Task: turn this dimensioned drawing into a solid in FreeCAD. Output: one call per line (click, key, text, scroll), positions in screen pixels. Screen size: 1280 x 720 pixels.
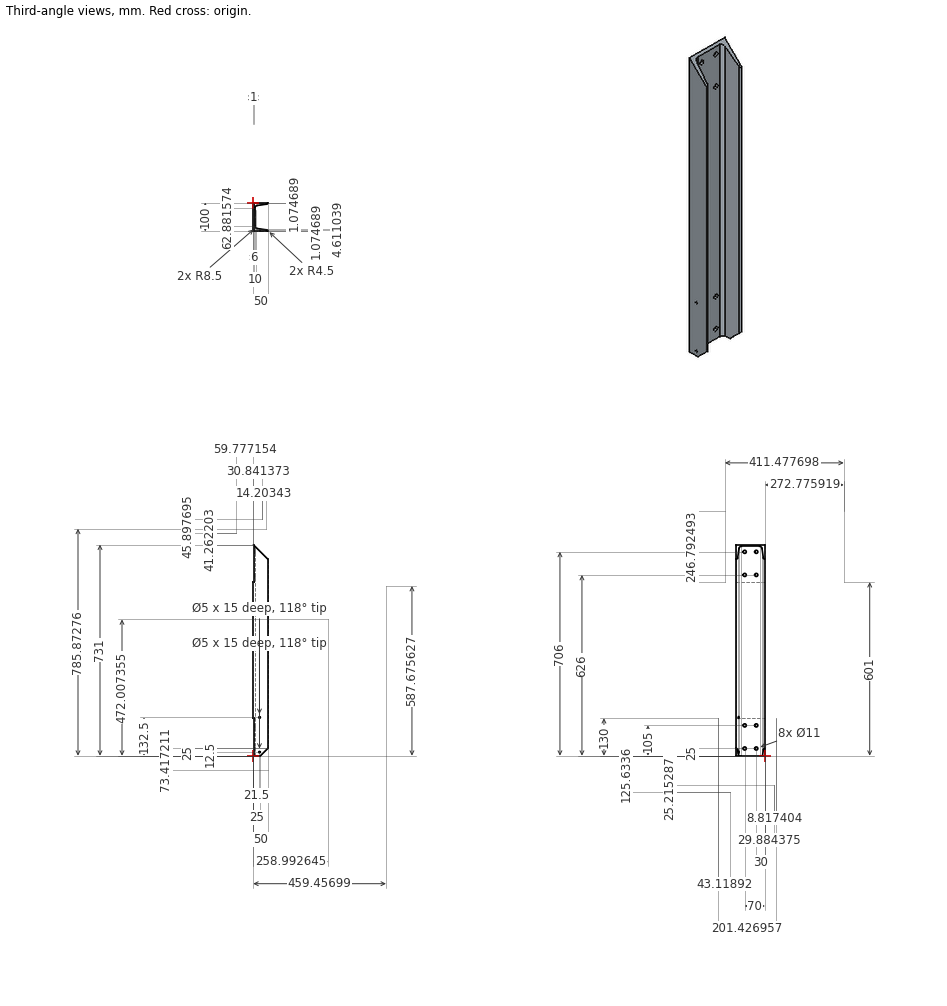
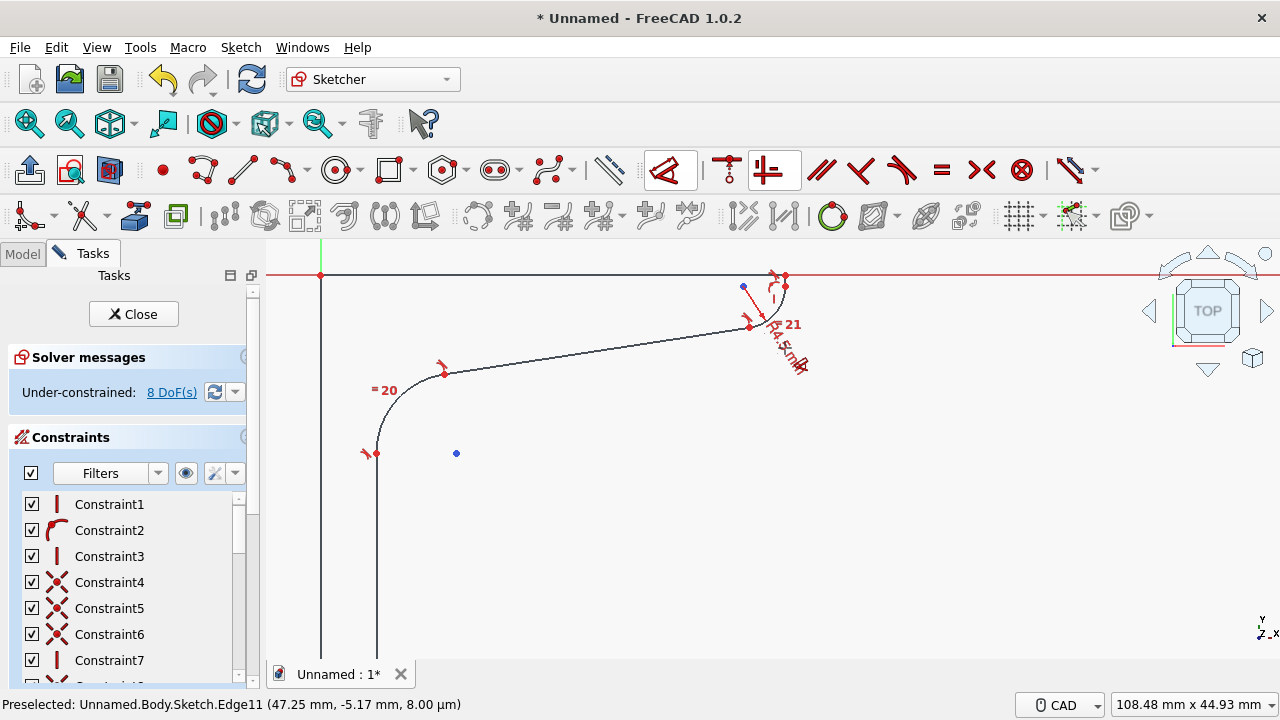
scroll(769, 322, down, 6)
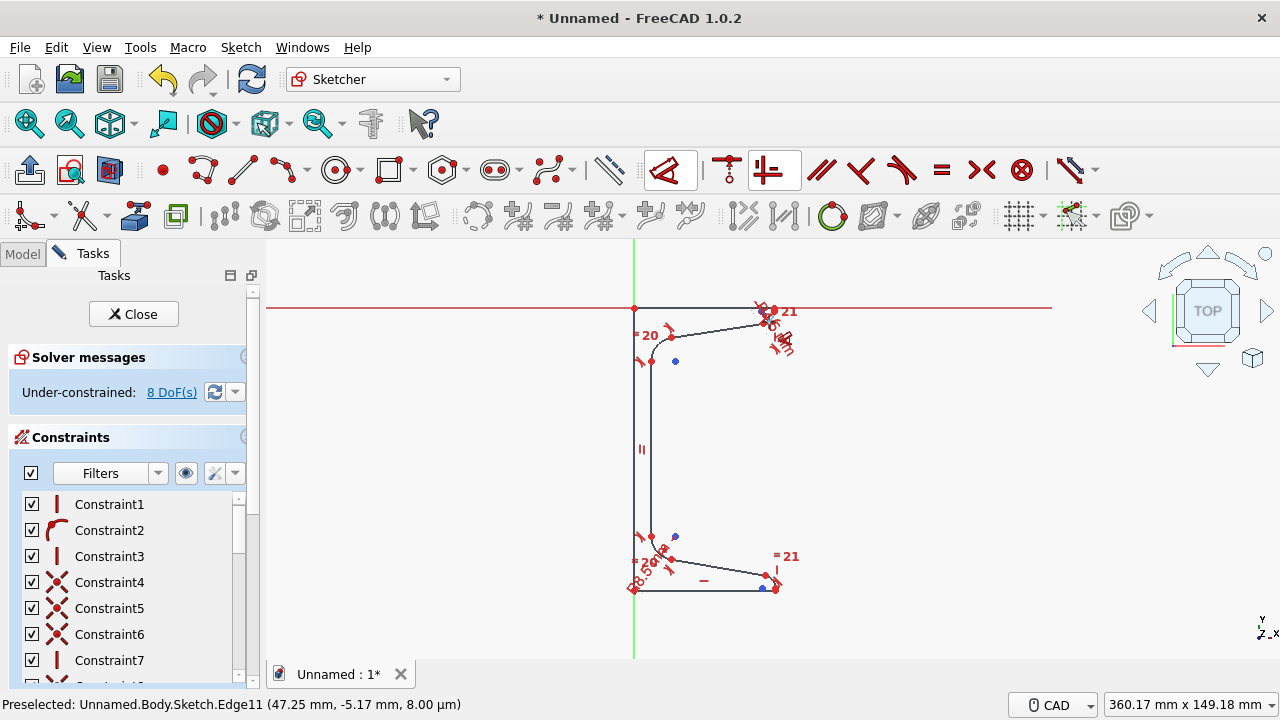
click(732, 308)
click(704, 274)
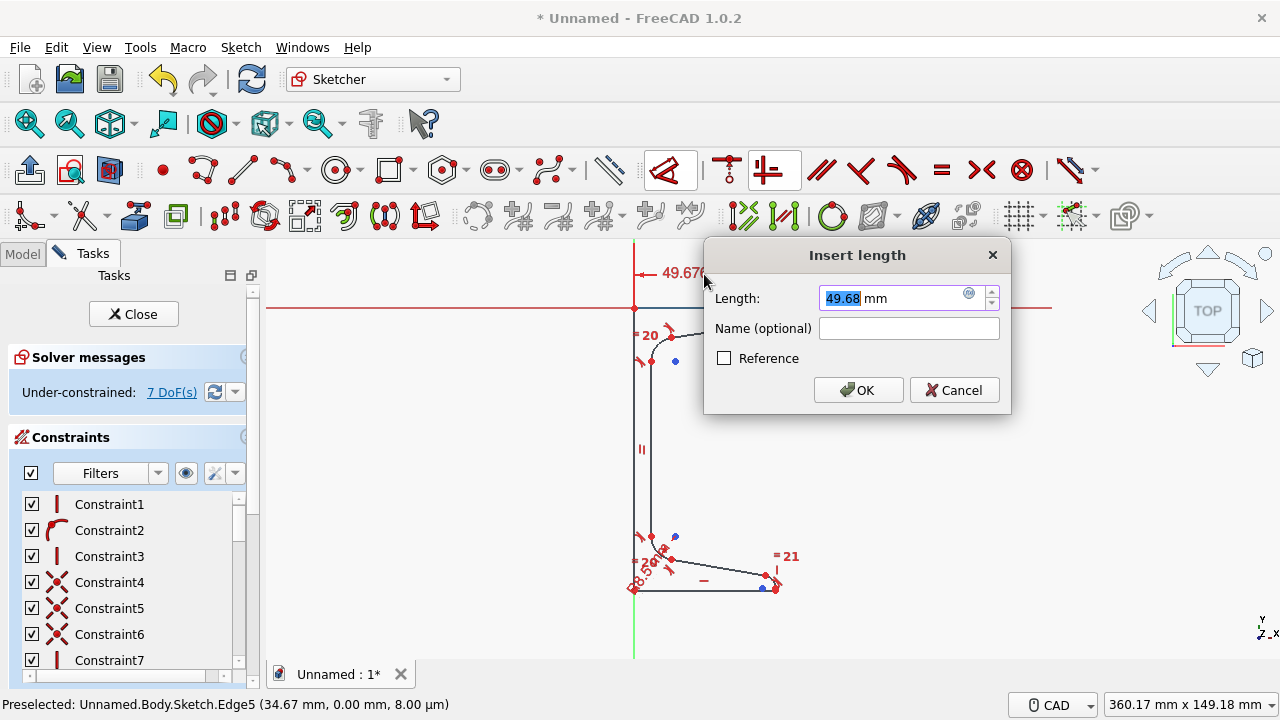
text(50)
key(Return)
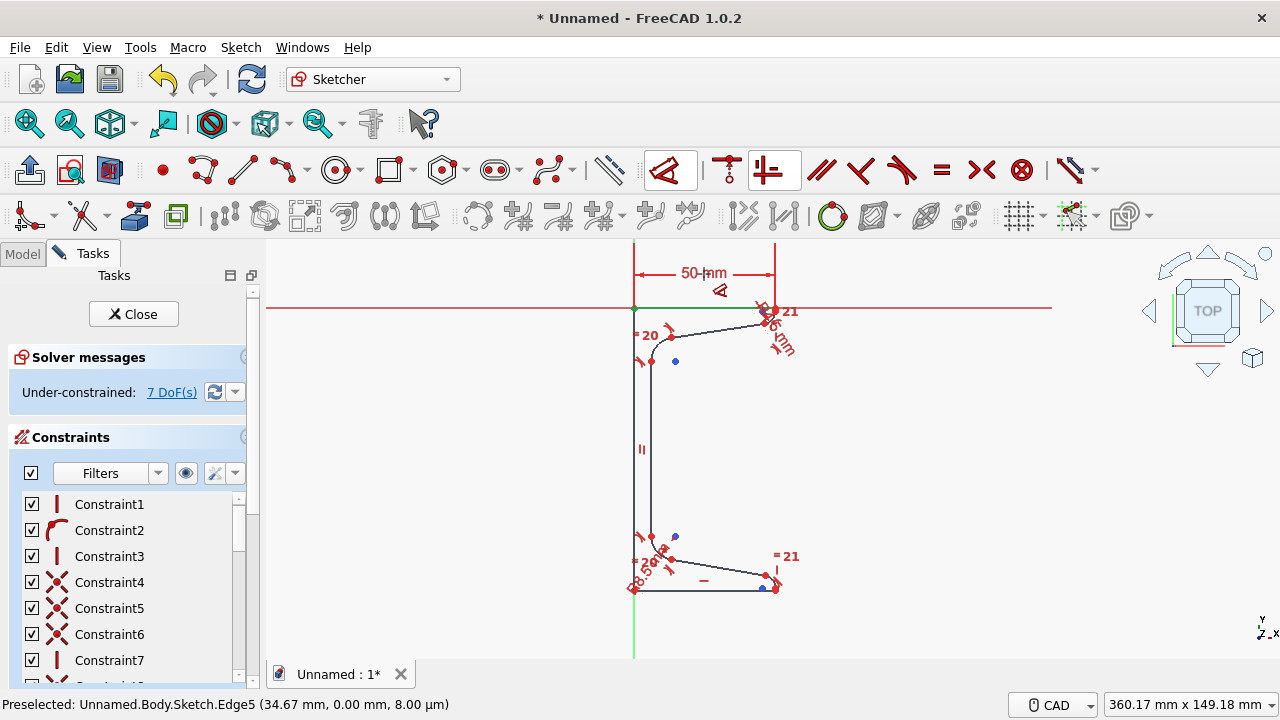
click(677, 591)
click(705, 625)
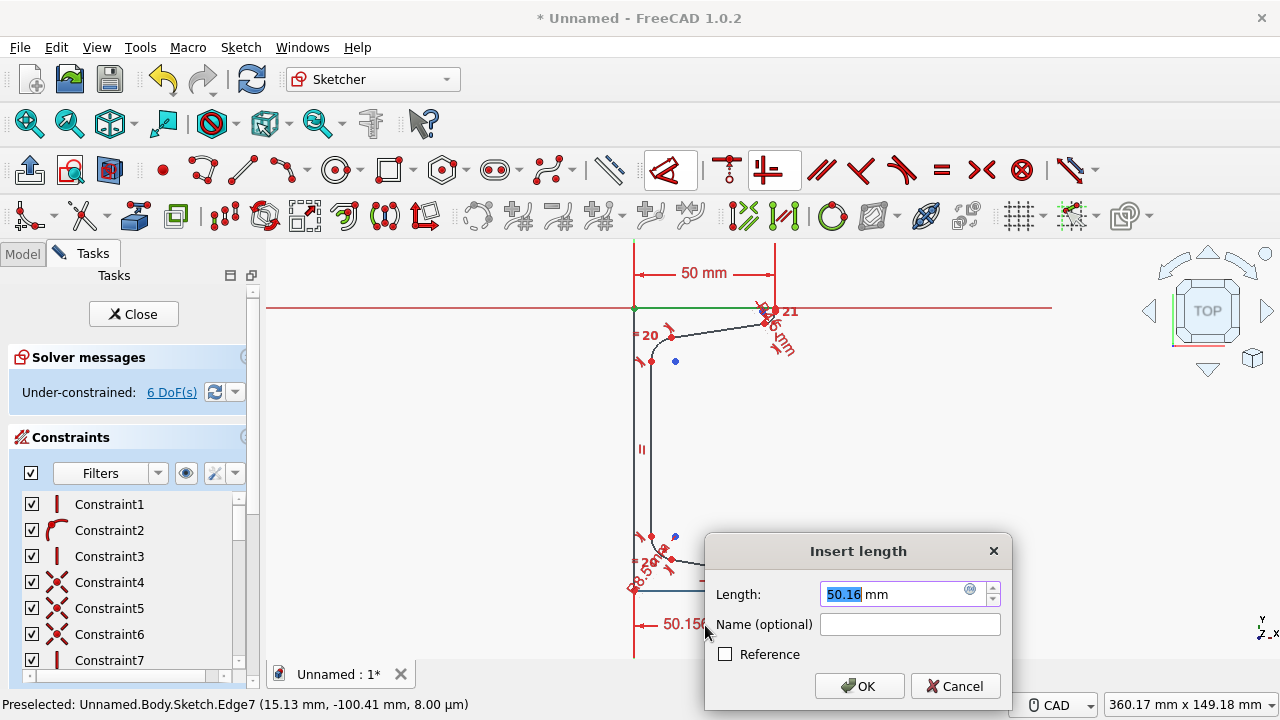
text(50)
key(Return)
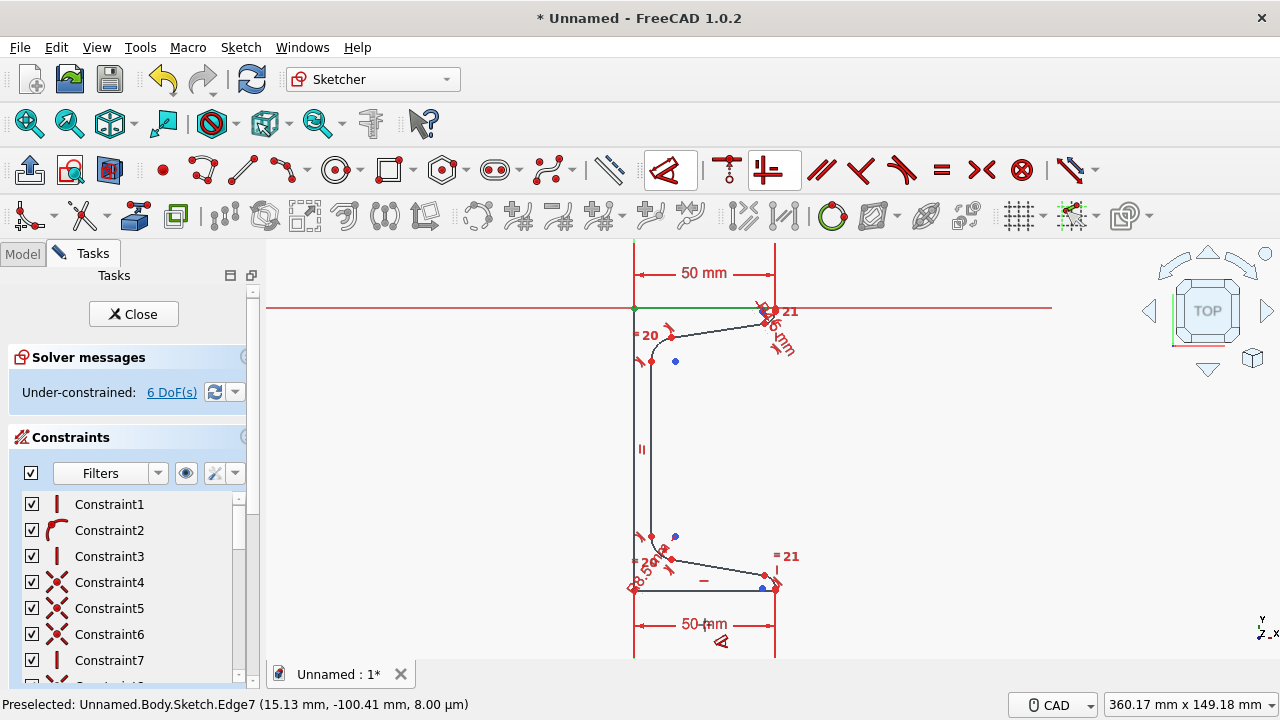
scroll(651, 536, up, 5)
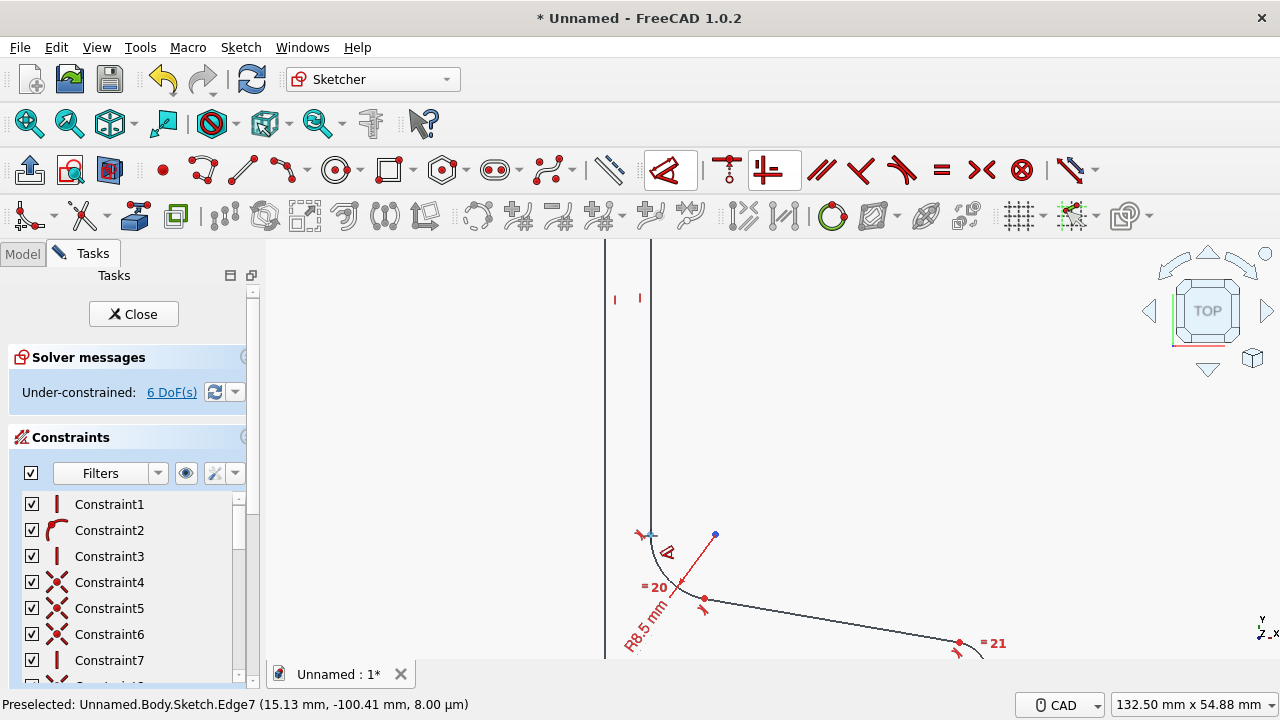
click(651, 535)
click(628, 569)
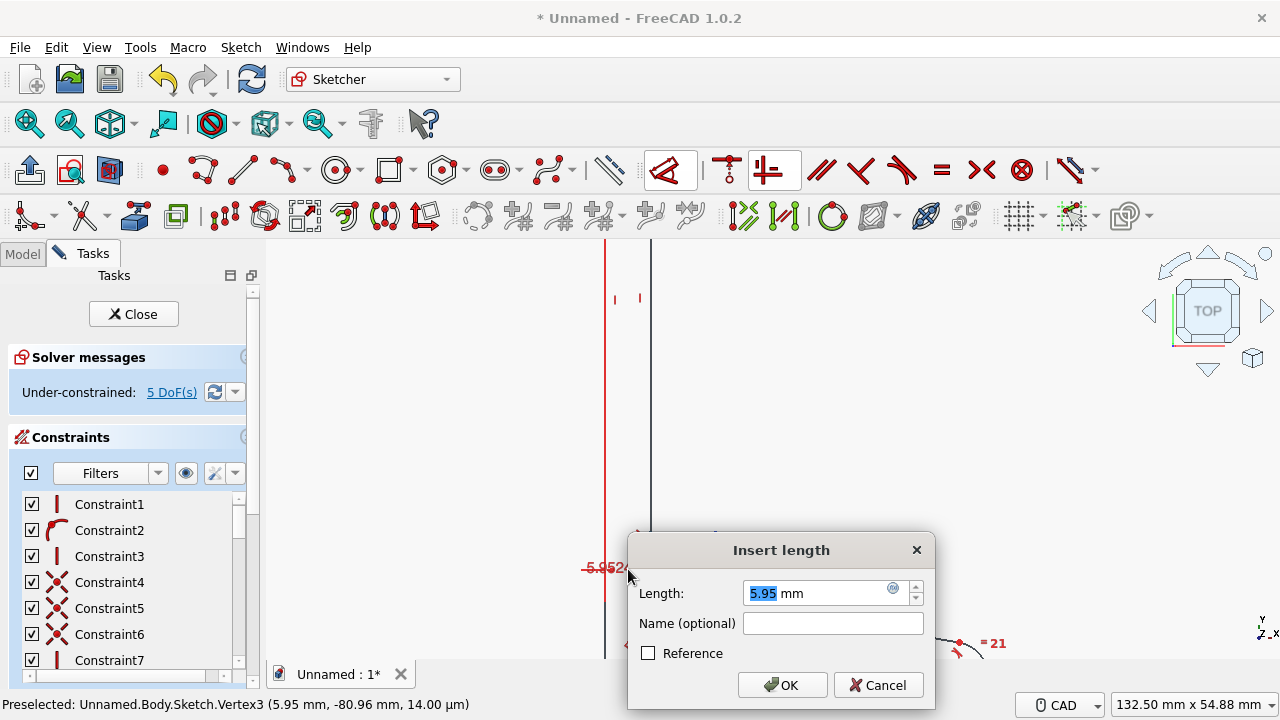
text(6)
key(Return)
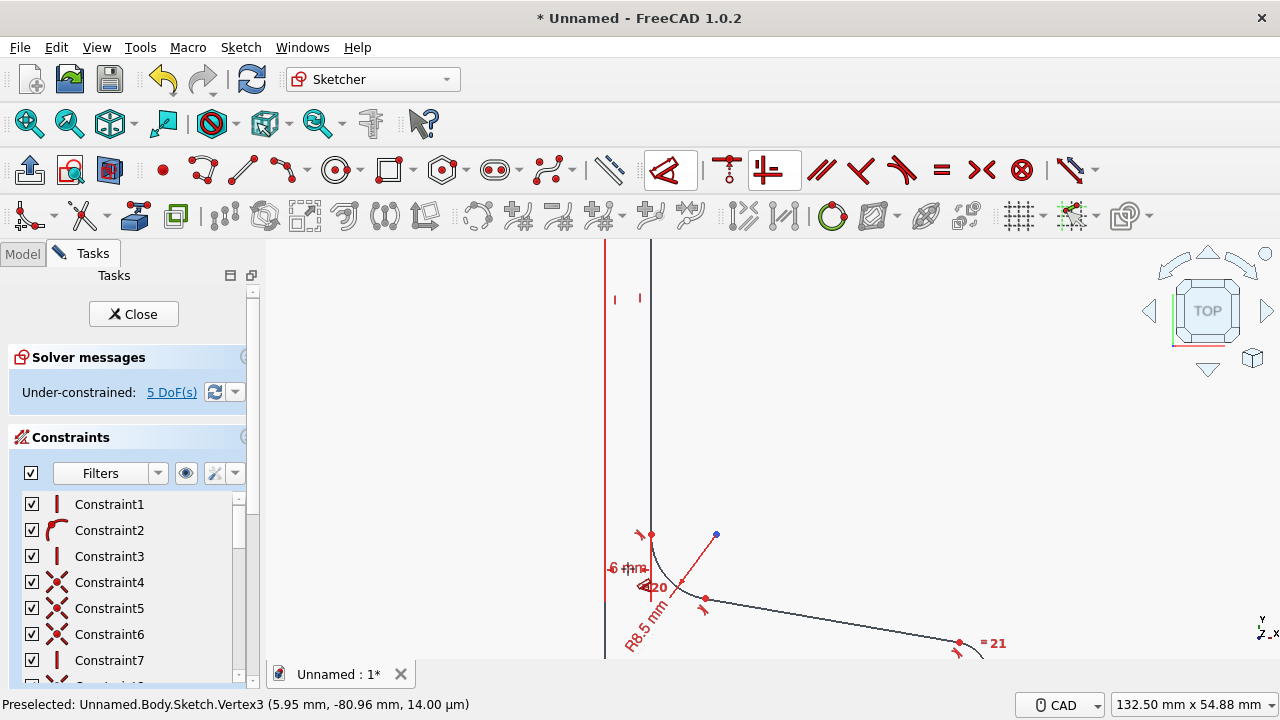
click(605, 453)
click(571, 449)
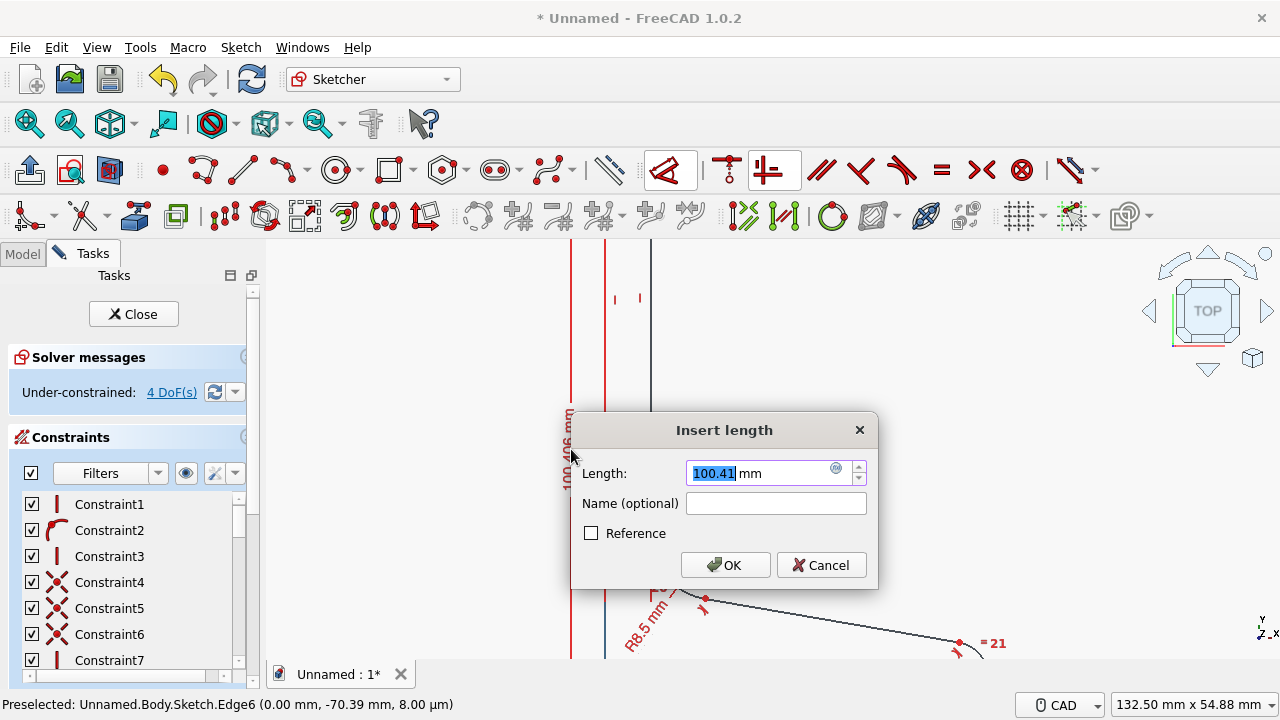
text(100)
key(Return)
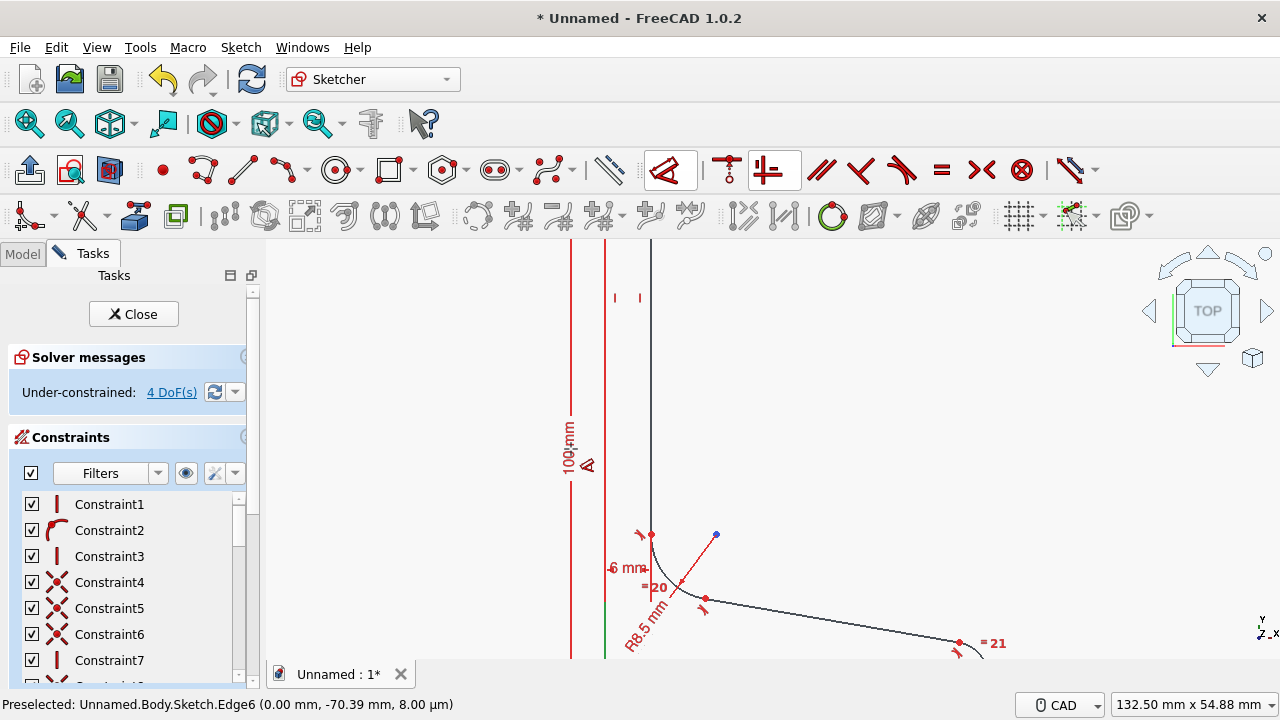
scroll(651, 537, down, 5)